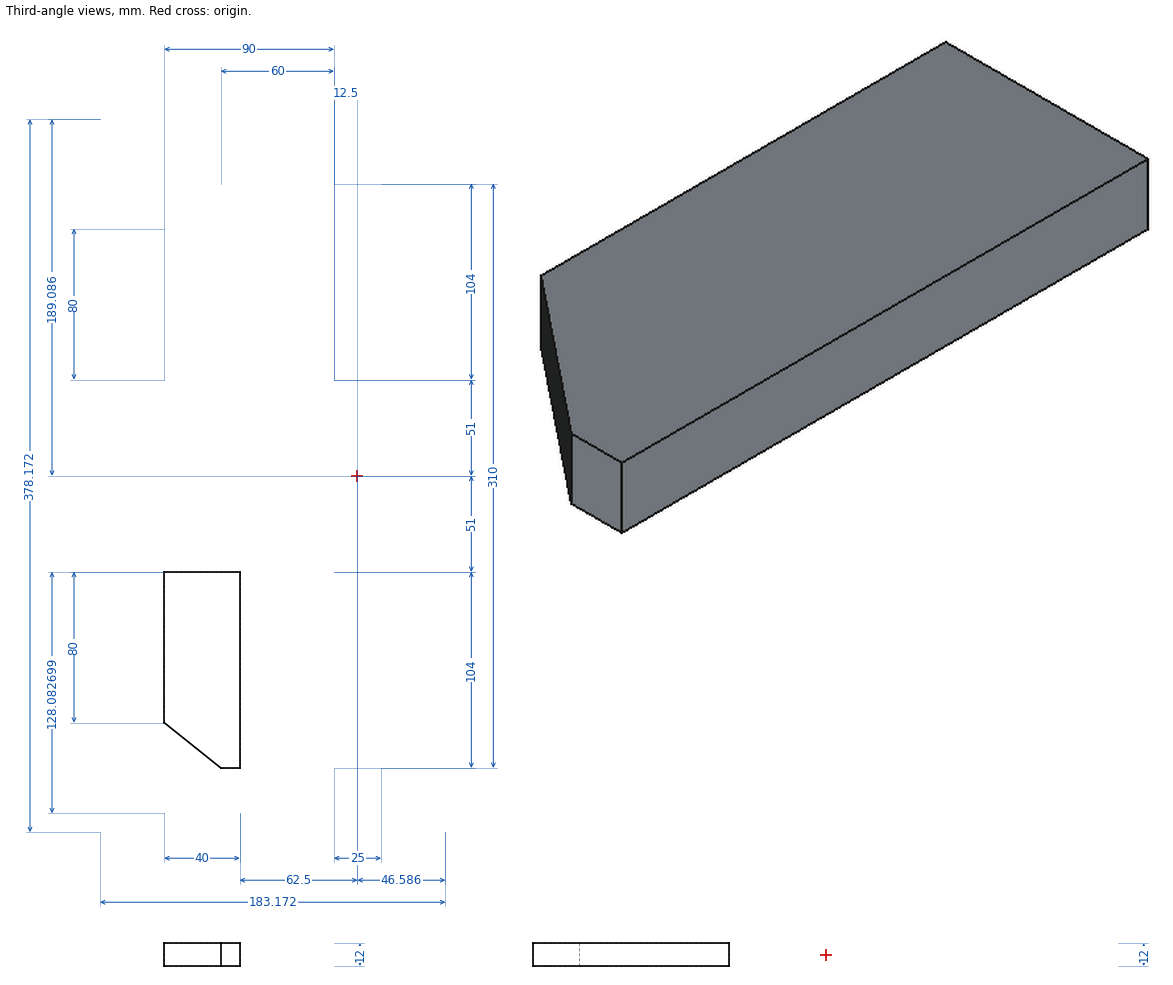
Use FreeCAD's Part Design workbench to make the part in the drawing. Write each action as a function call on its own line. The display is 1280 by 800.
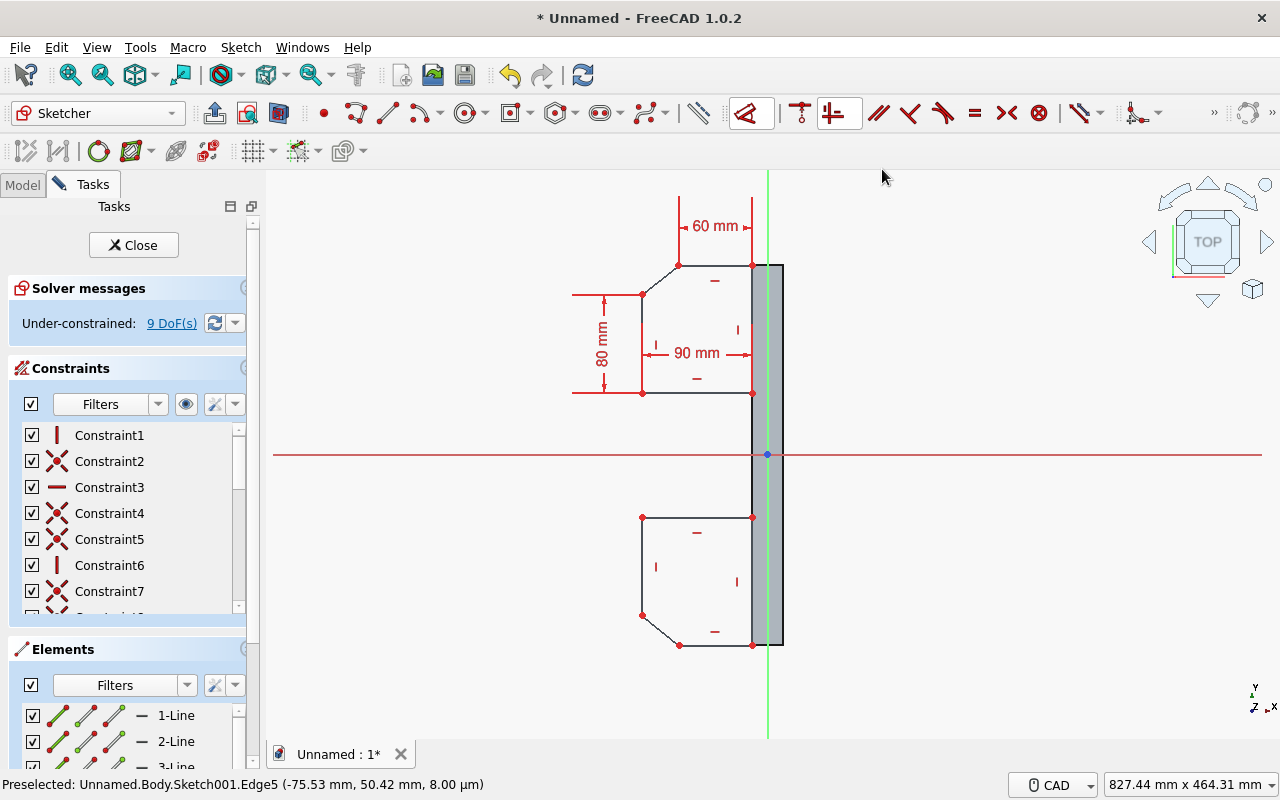
click(719, 518)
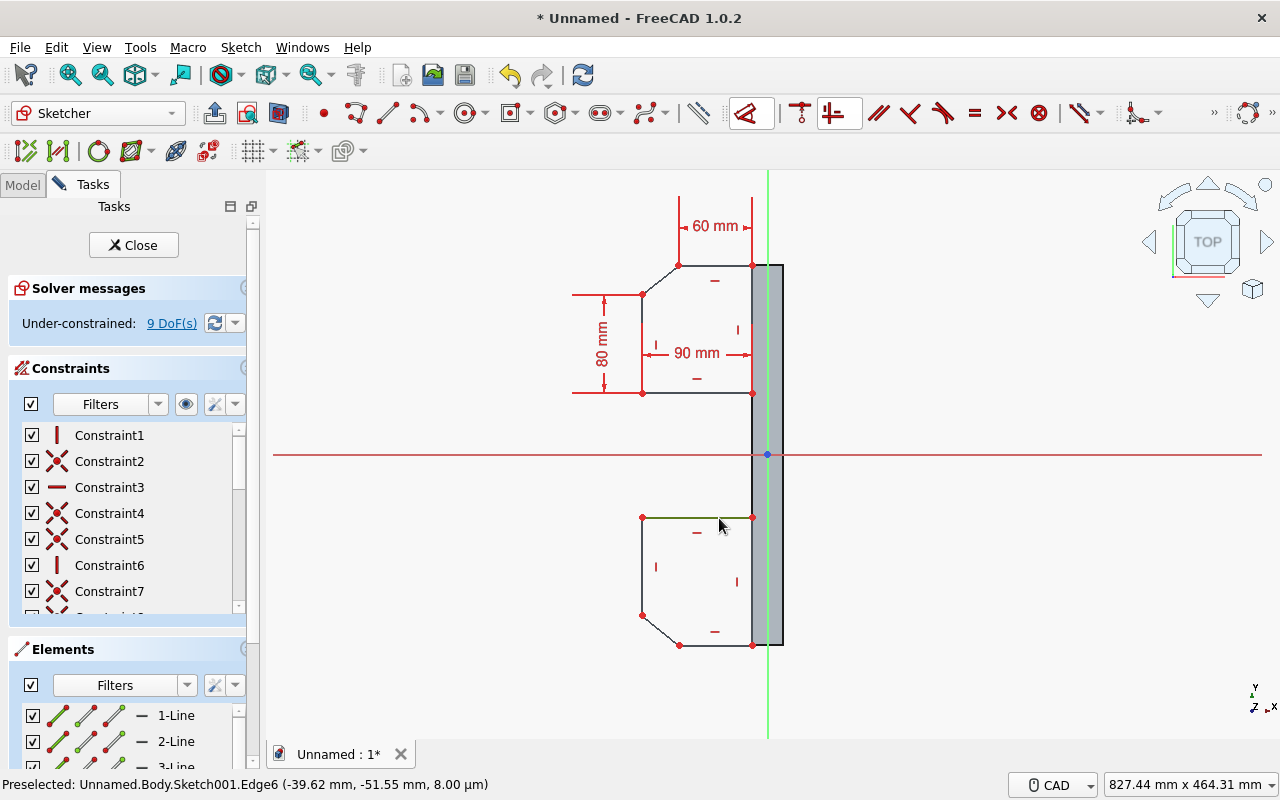
click(768, 114)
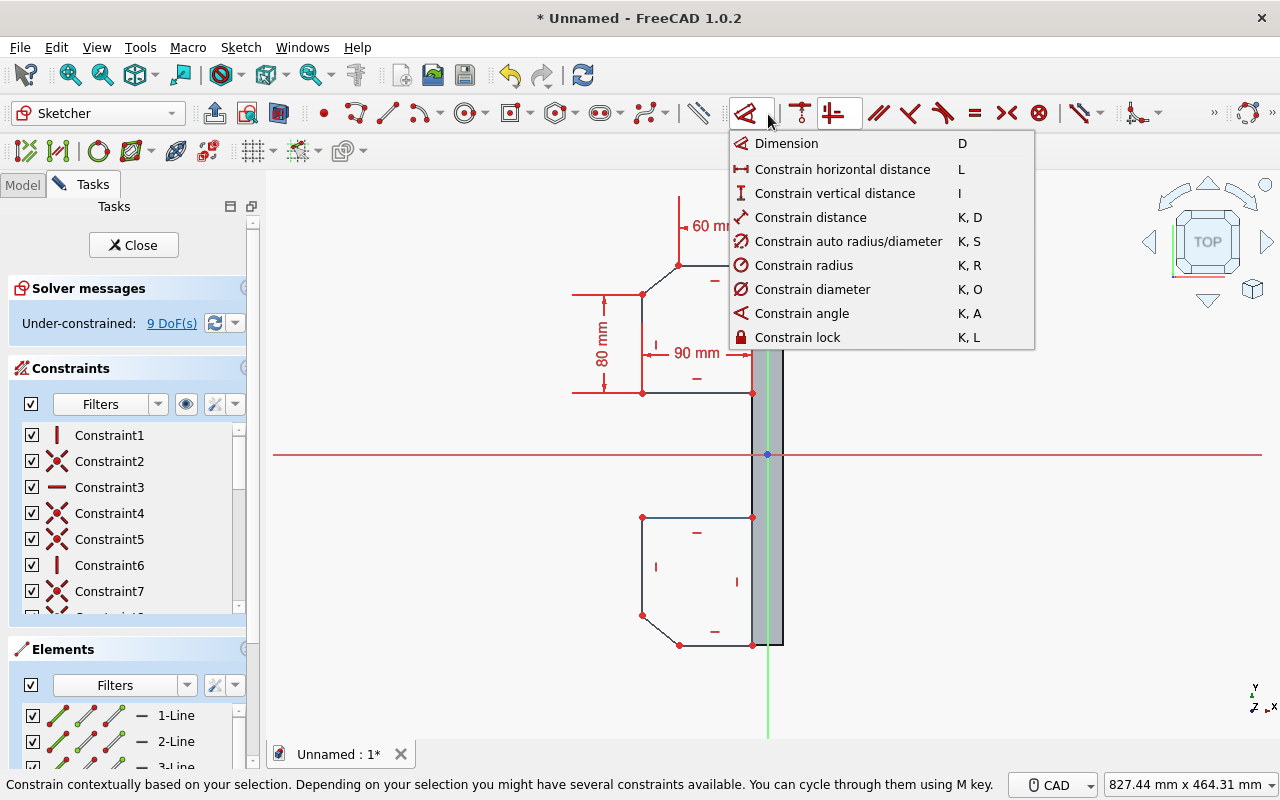
click(882, 169)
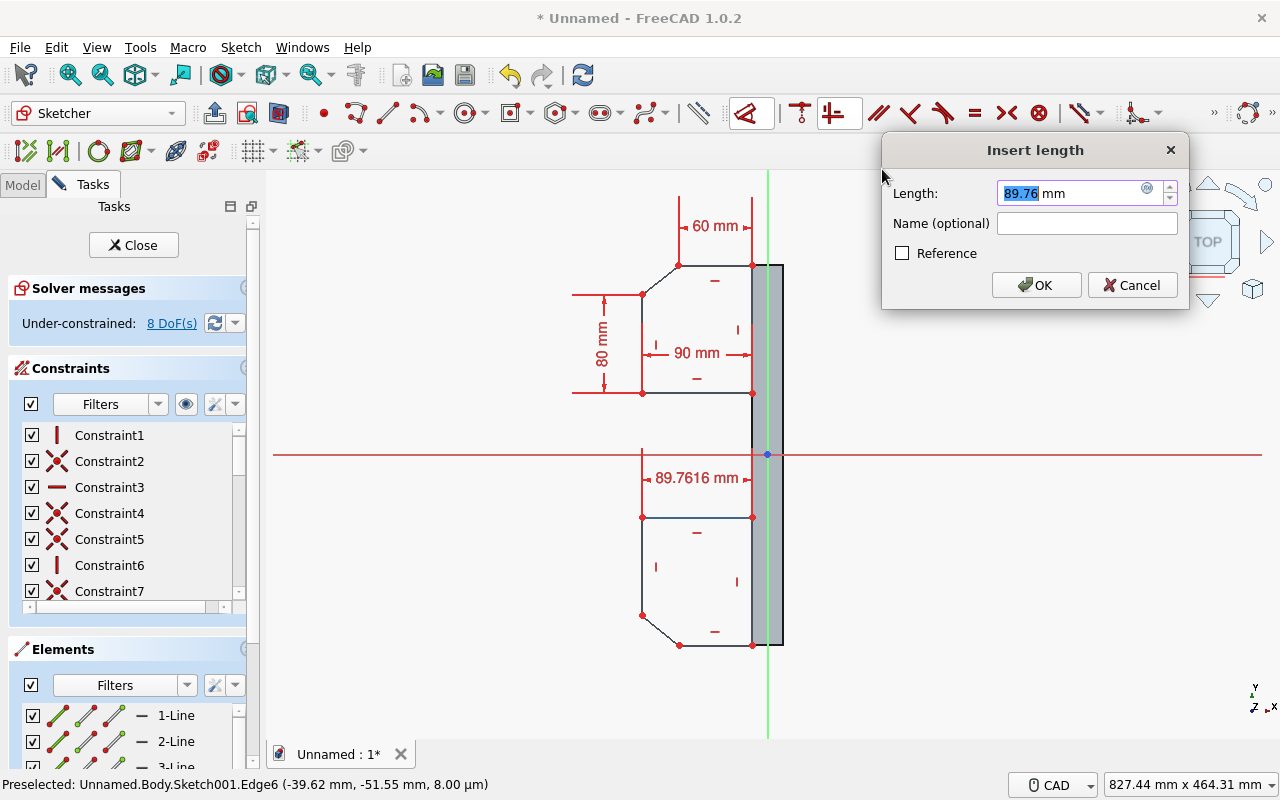
text(90)
key(Return)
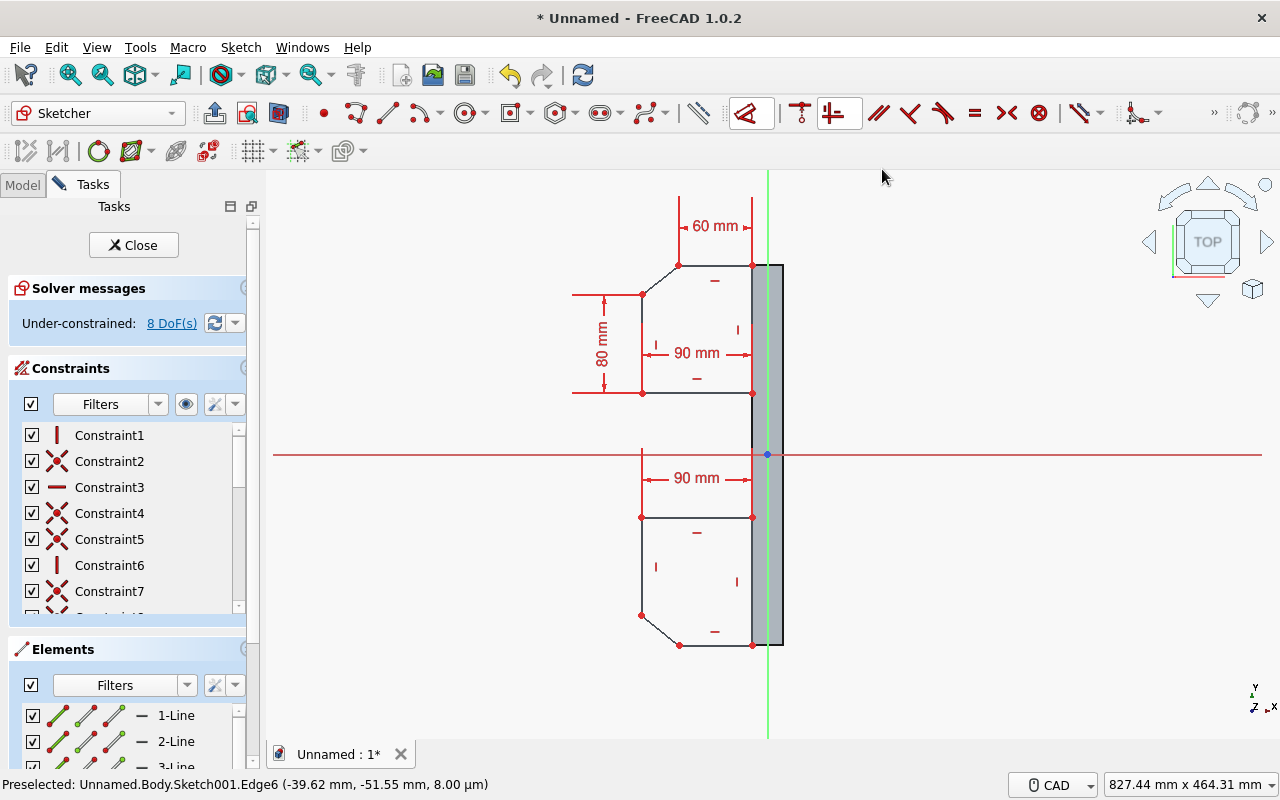
click(642, 547)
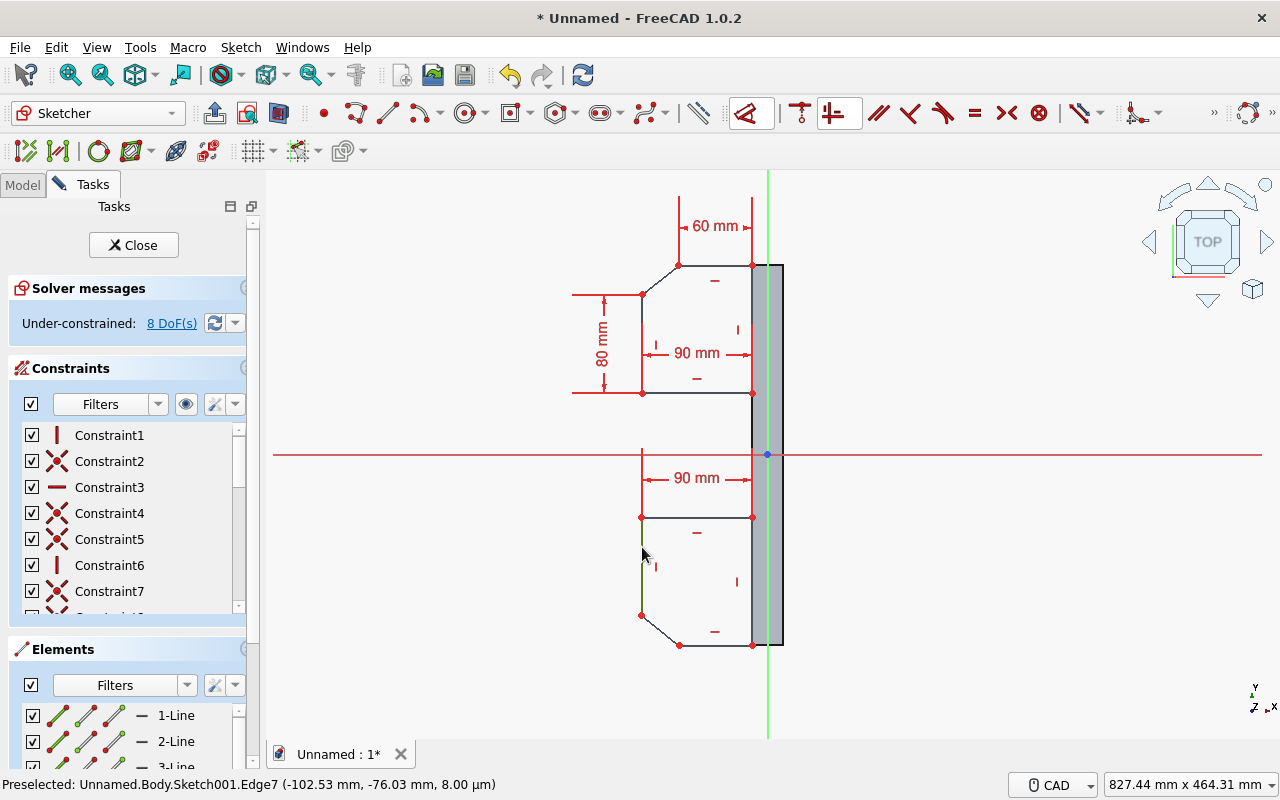
click(768, 114)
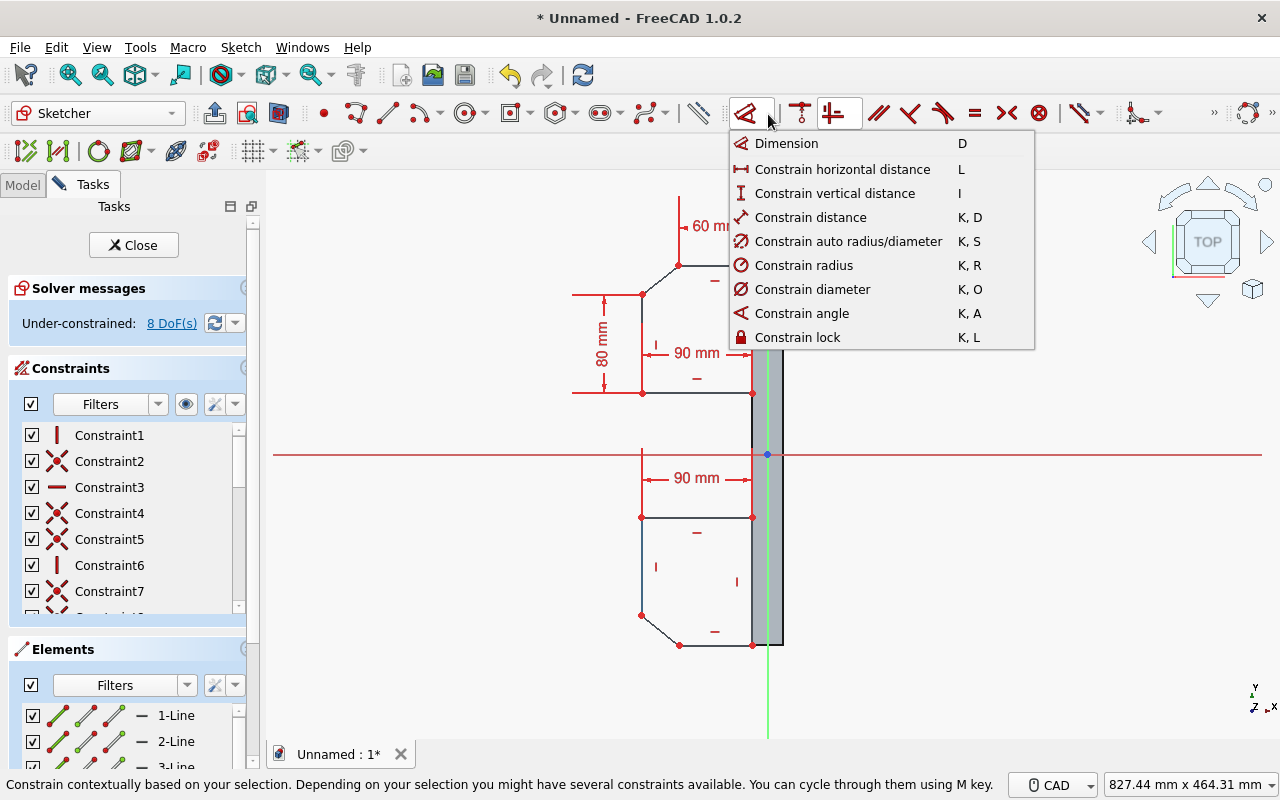
click(882, 193)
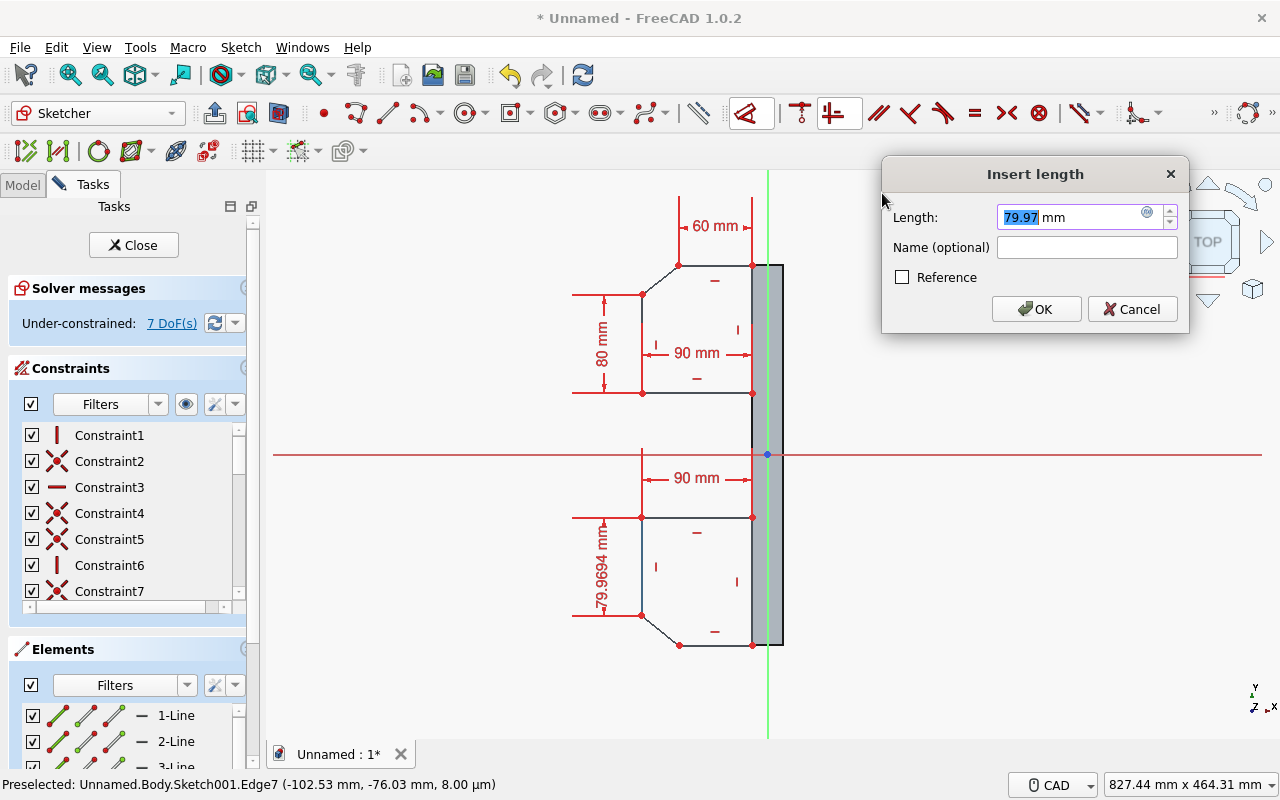
text(80)
key(Return)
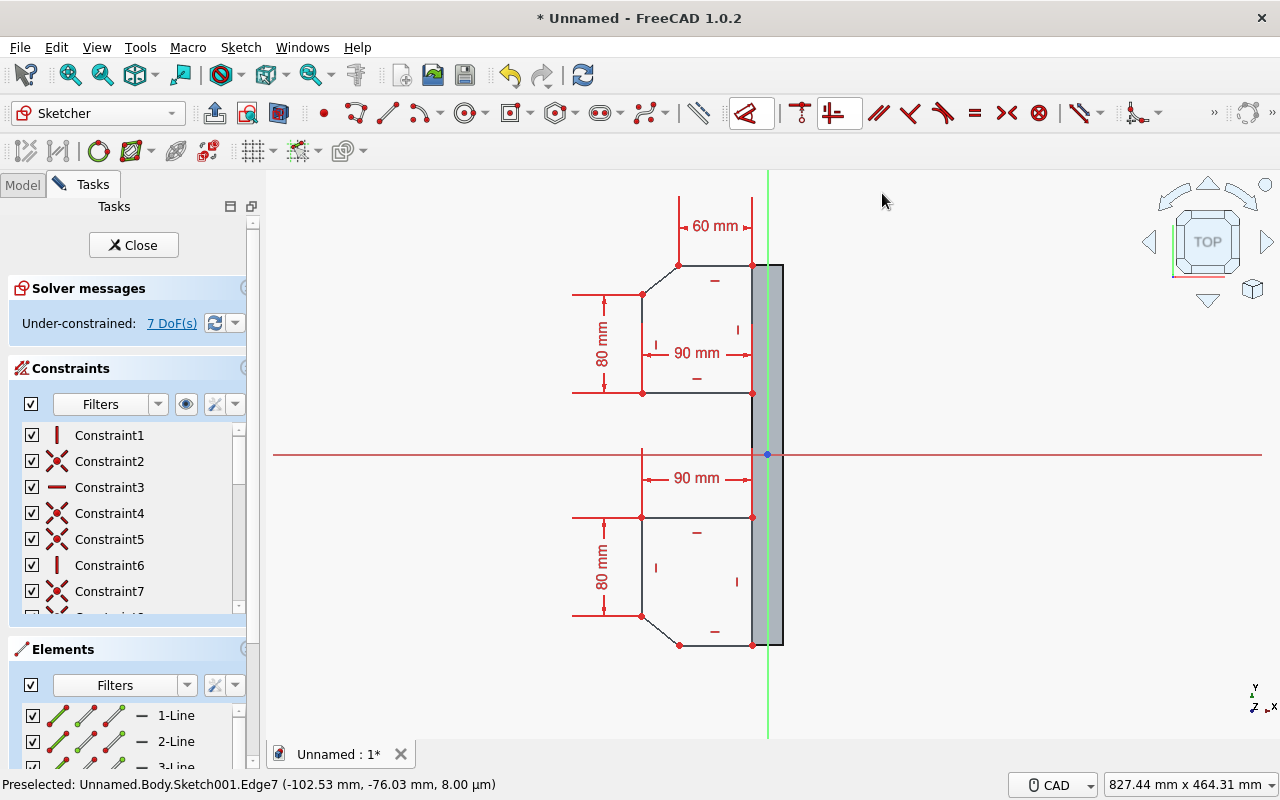
click(701, 646)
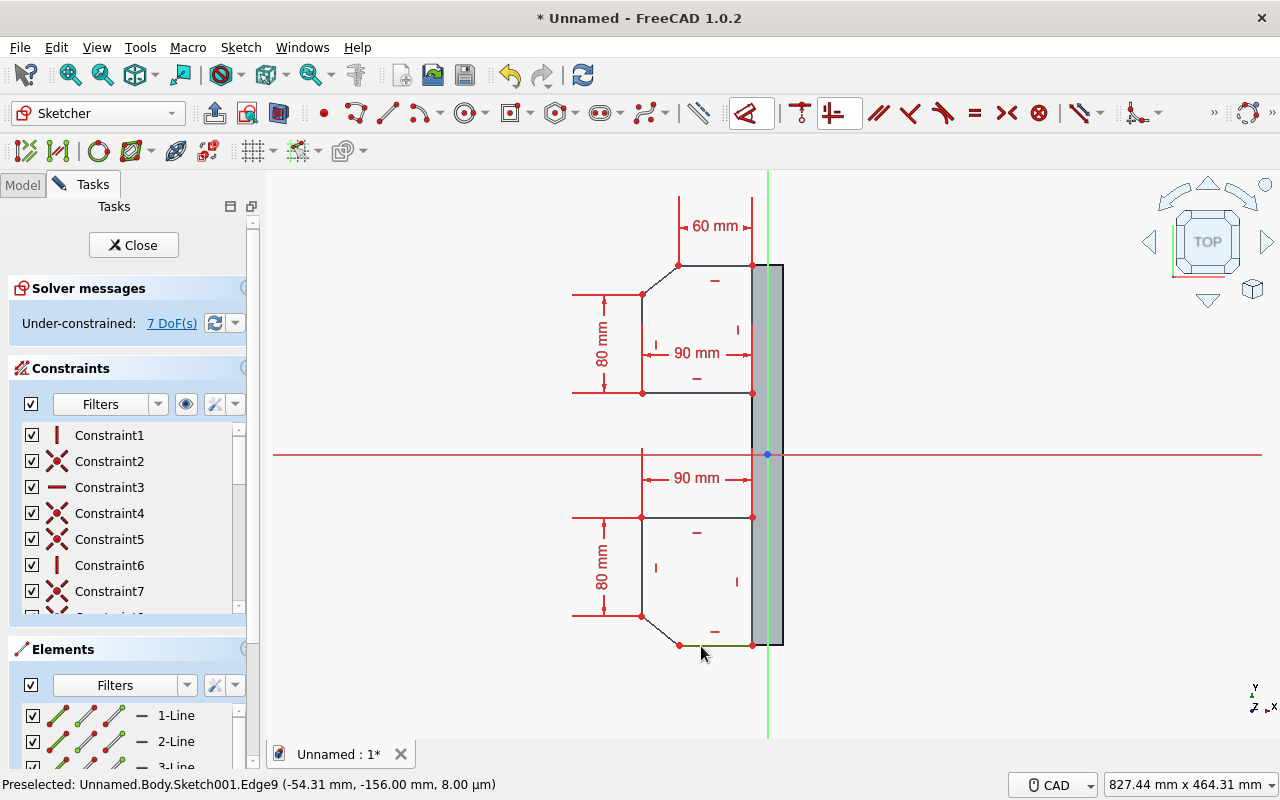
click(768, 114)